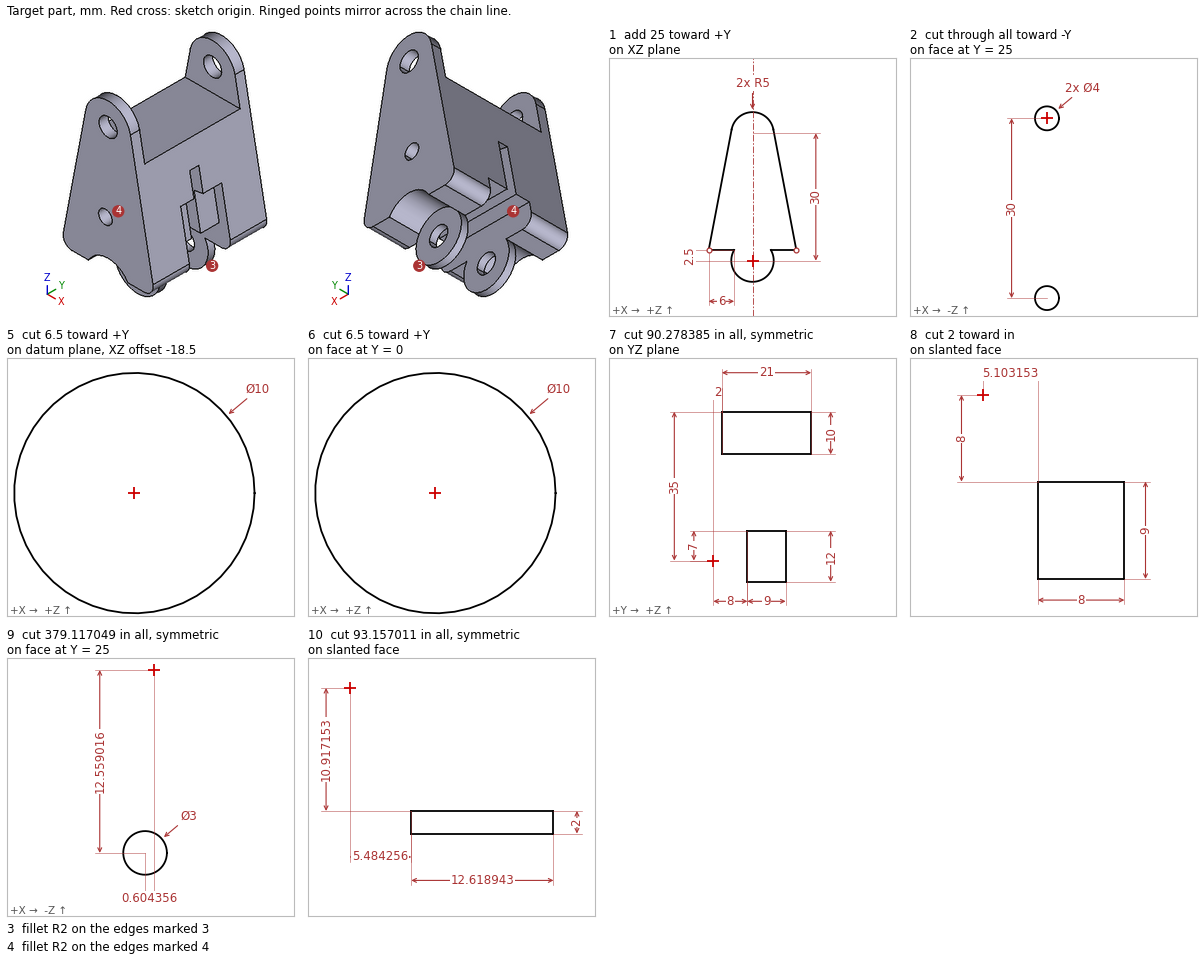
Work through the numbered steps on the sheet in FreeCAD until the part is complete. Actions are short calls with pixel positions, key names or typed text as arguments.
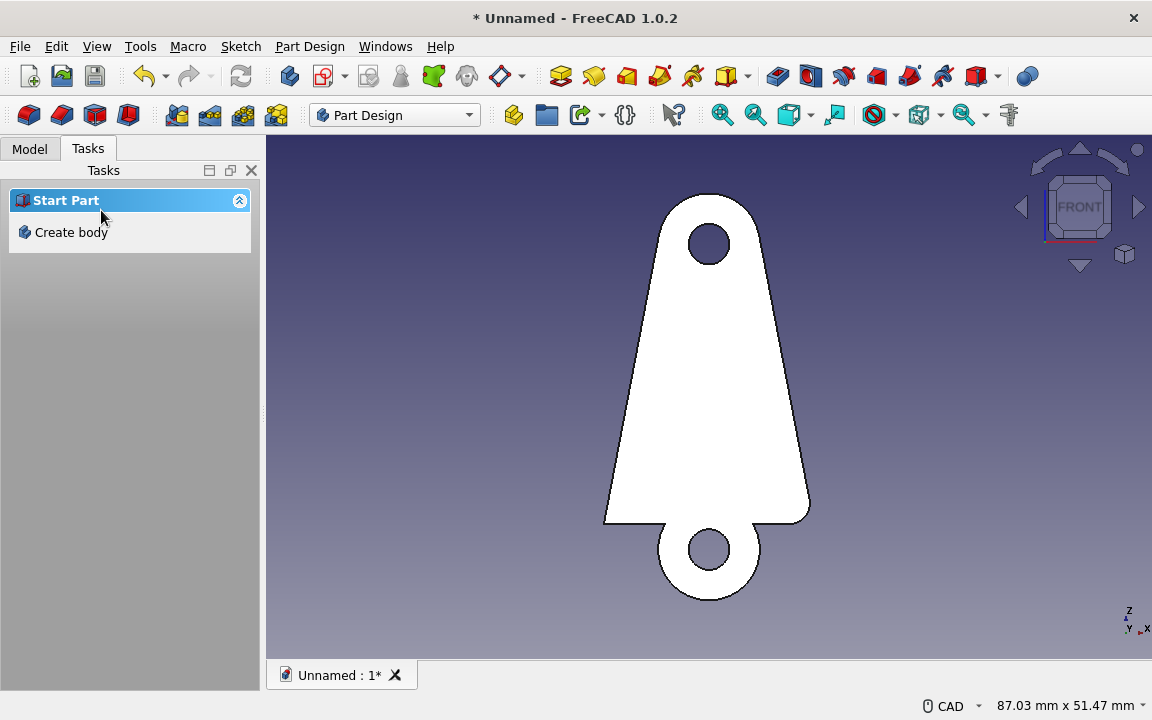
key(3)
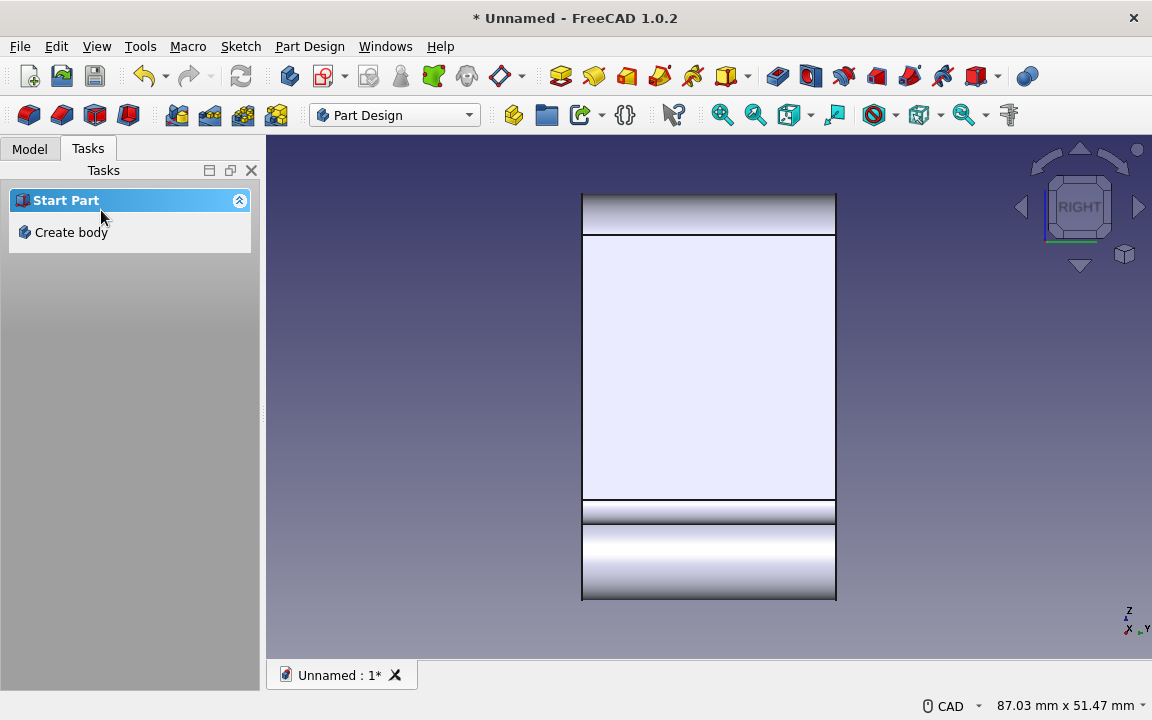
key(5)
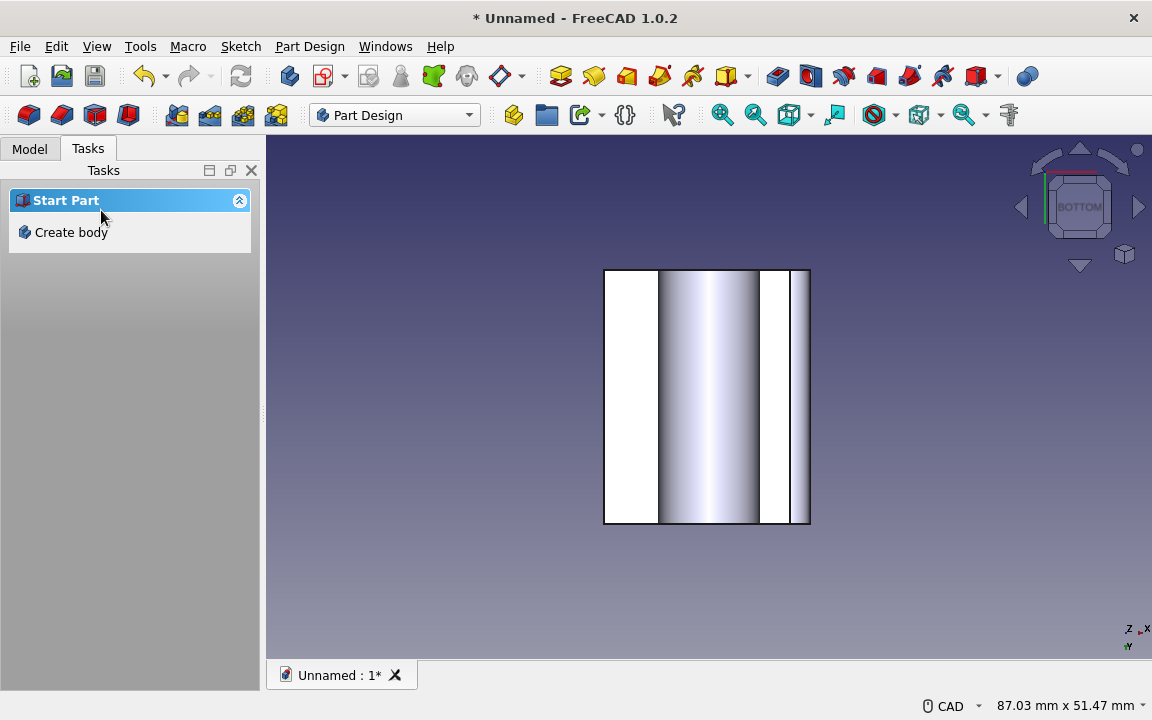
click(604, 396)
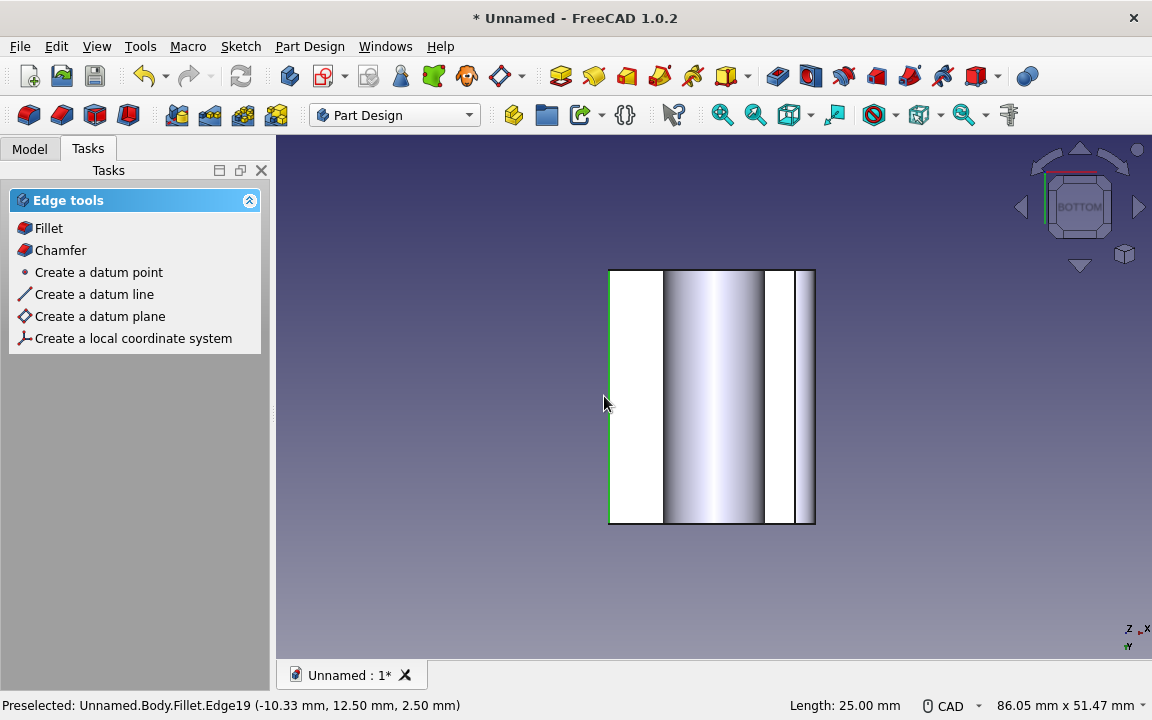
click(29, 116)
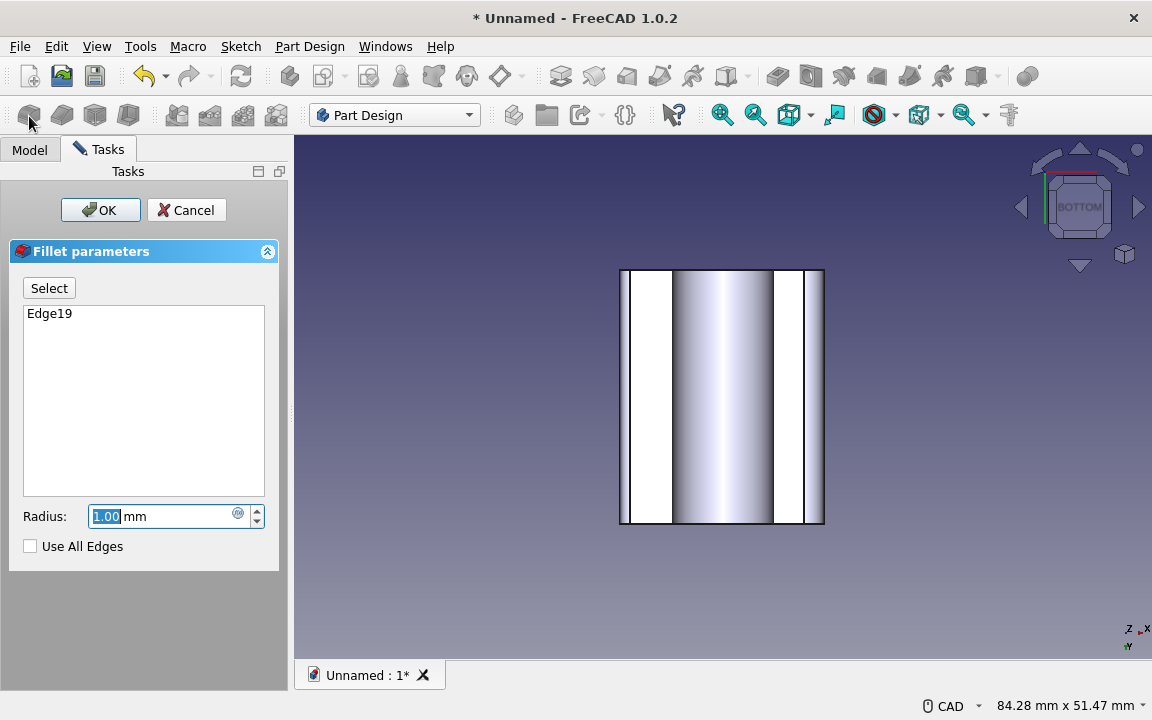
text(2)
key(Tab)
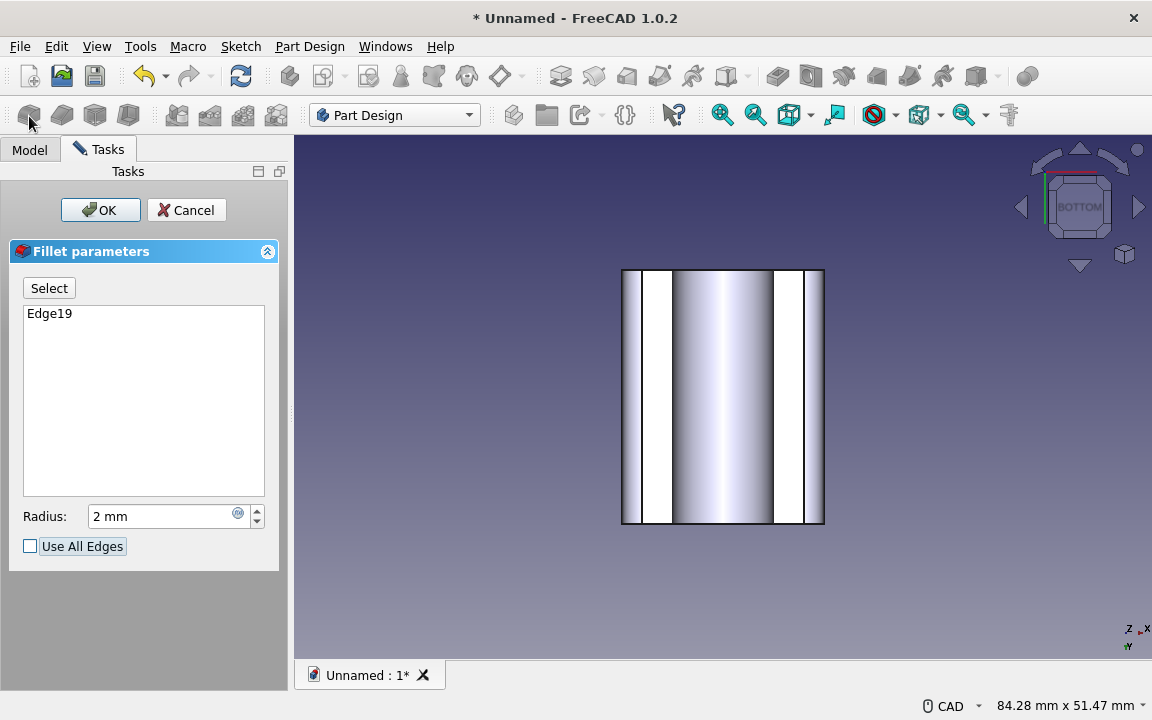
click(101, 210)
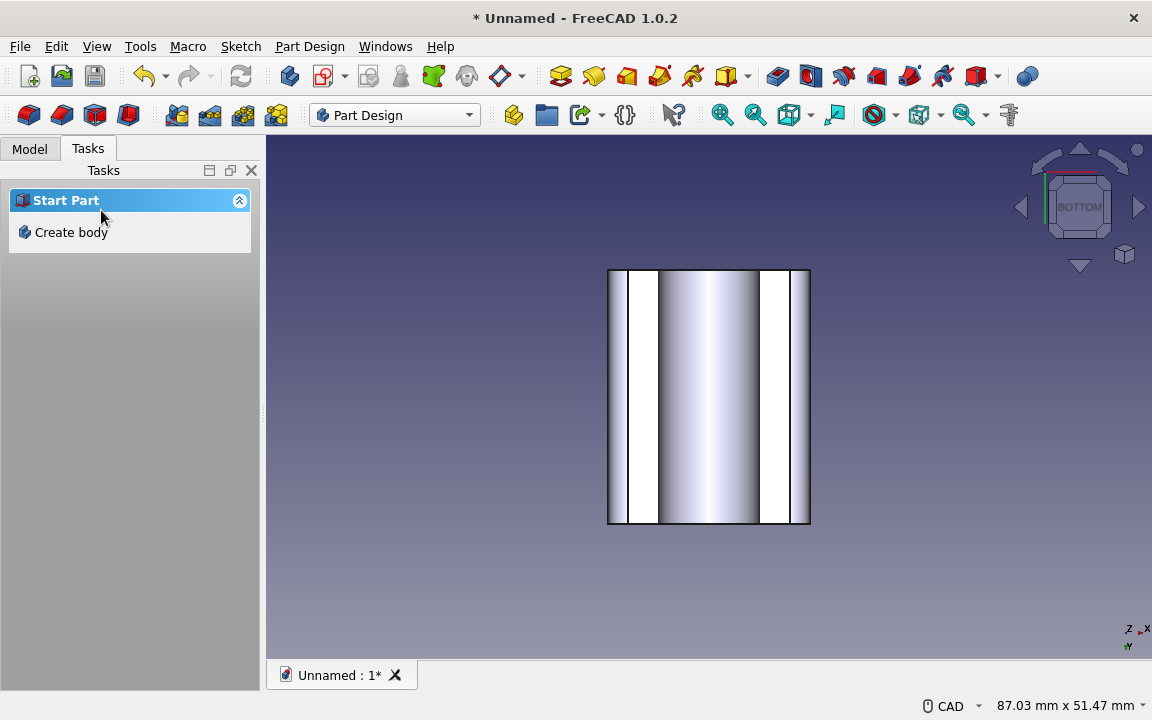
click(30, 148)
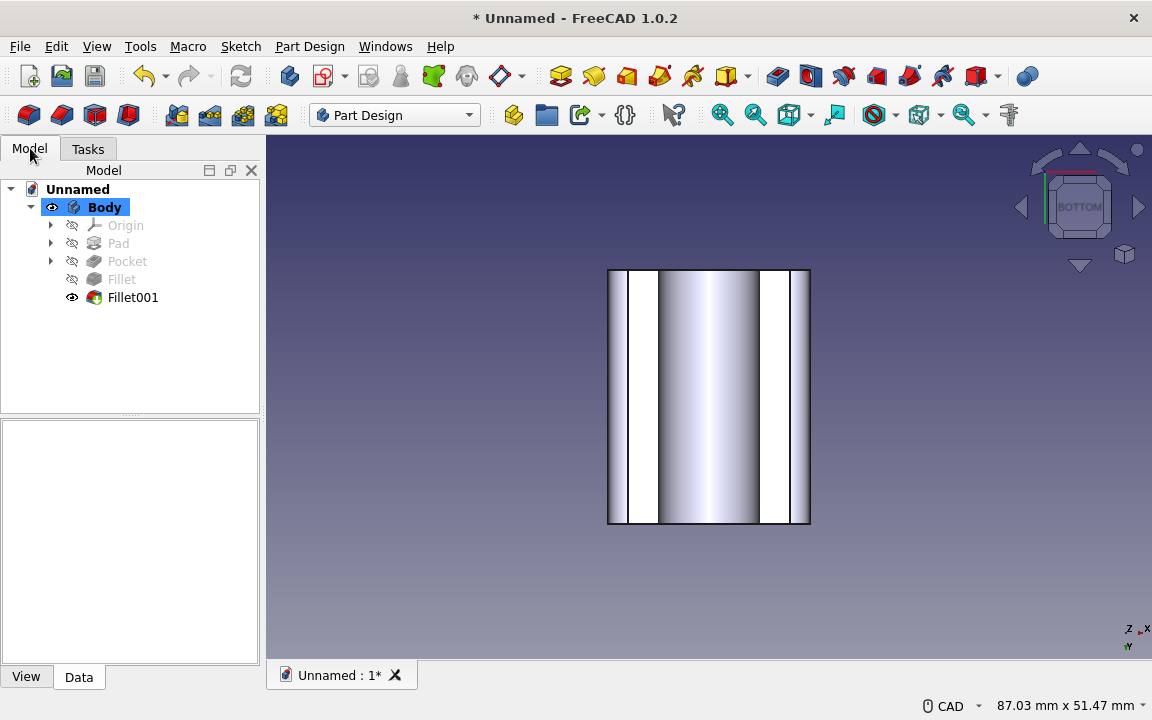
click(51, 225)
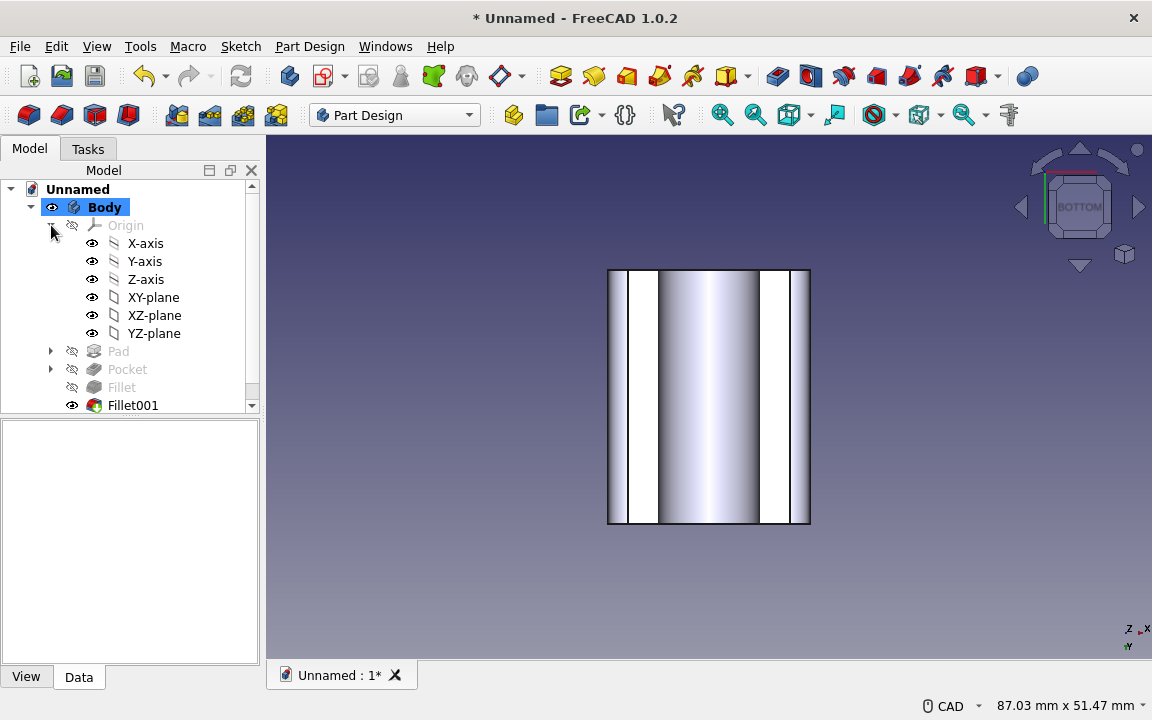
click(137, 315)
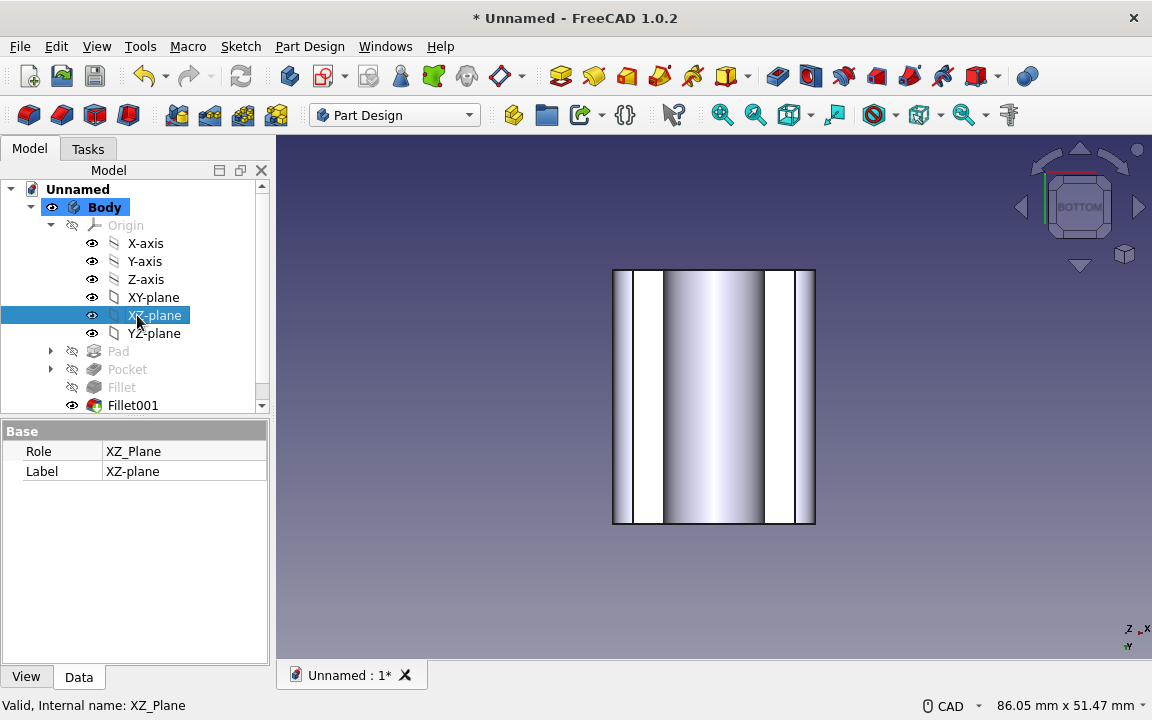
click(500, 76)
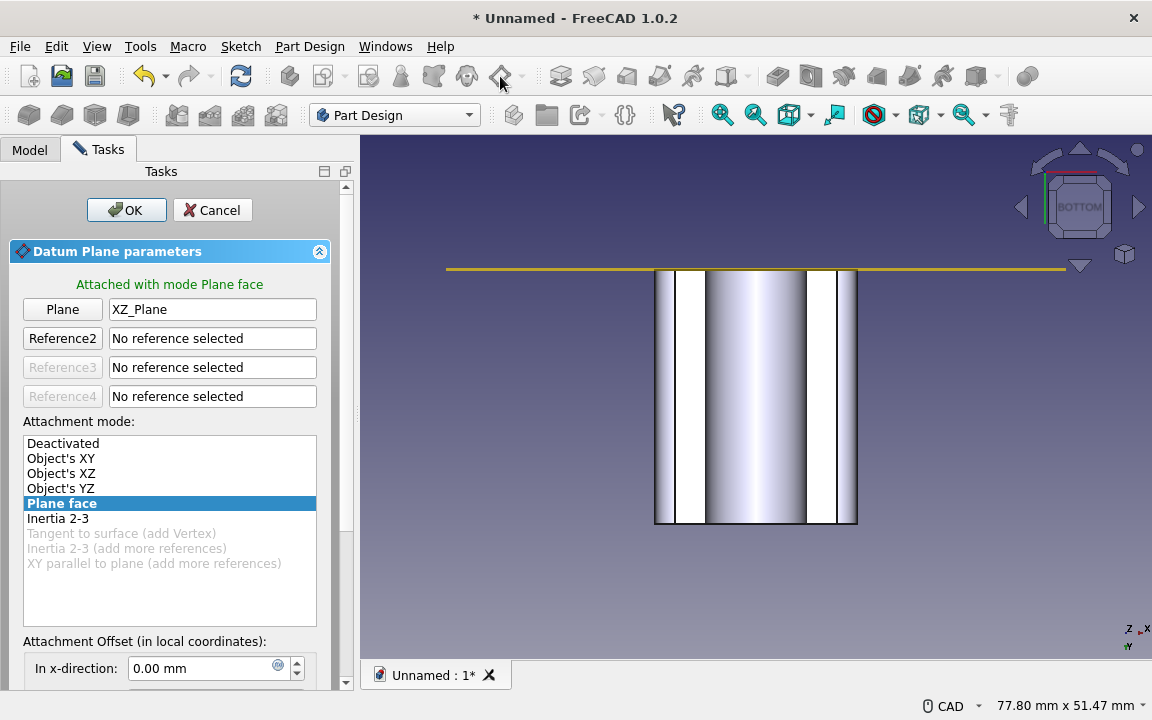
scroll(346, 436, down, 2)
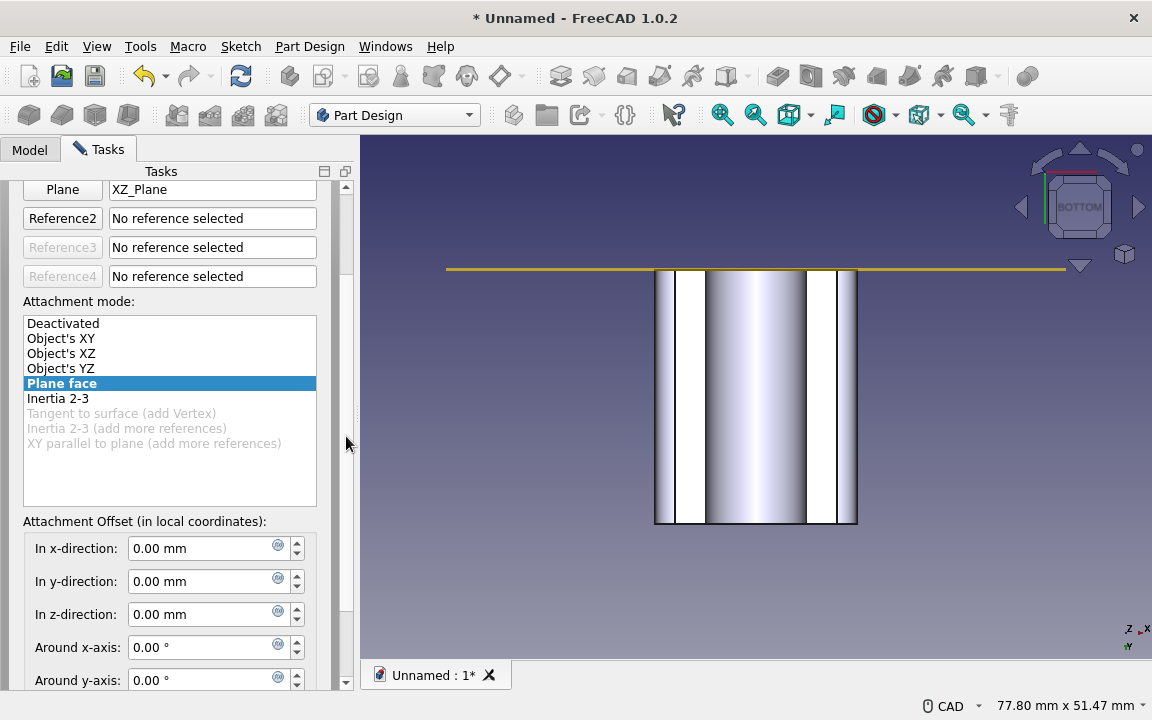
triple_click(210, 614)